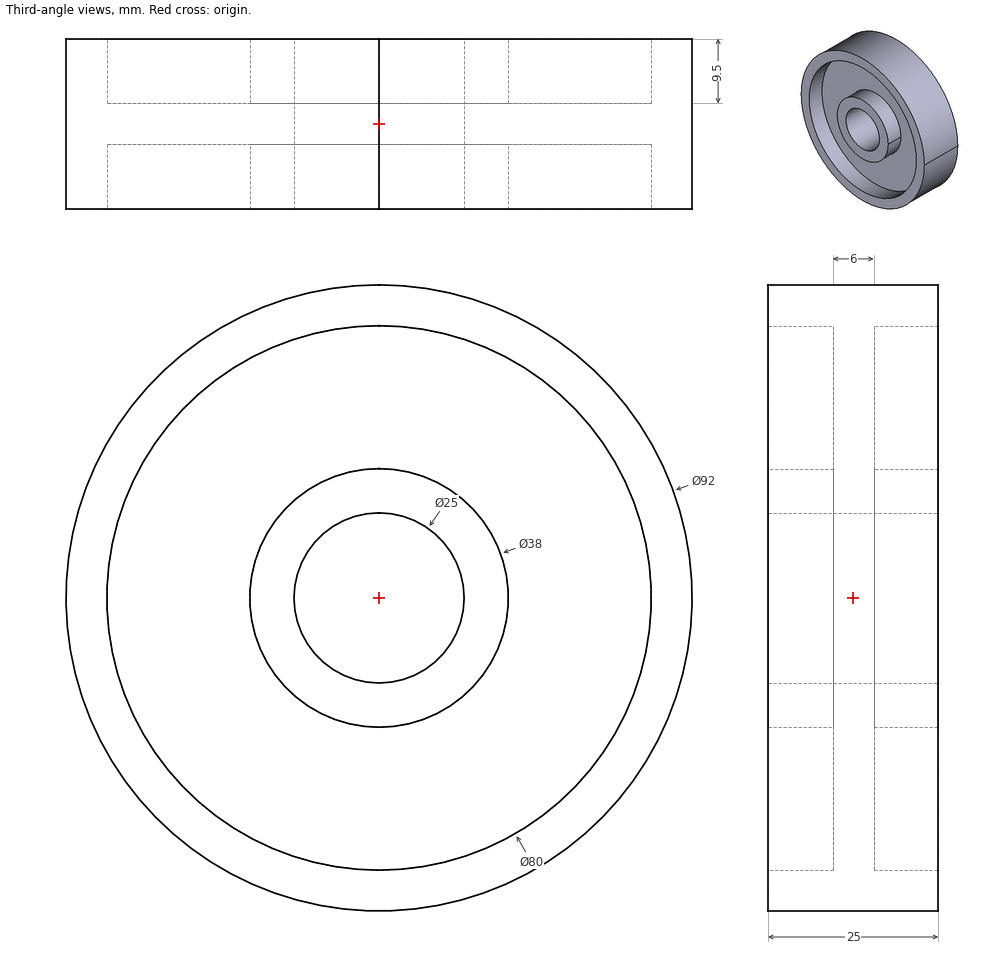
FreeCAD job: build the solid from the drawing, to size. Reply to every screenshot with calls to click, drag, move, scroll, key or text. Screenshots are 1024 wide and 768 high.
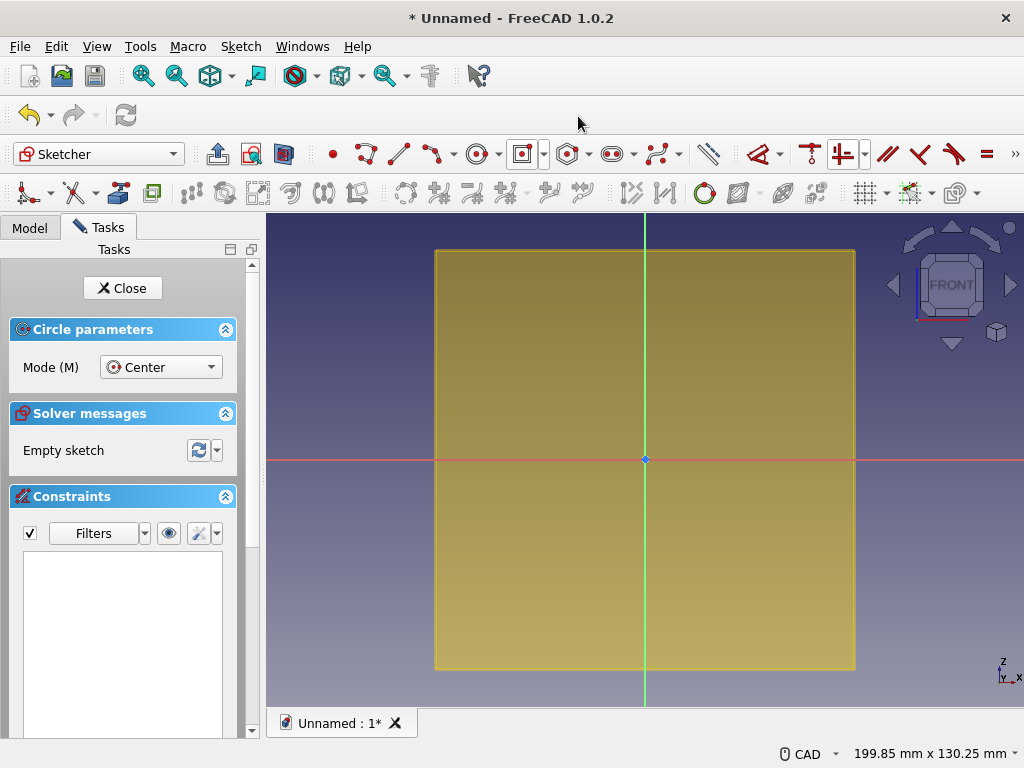
click(645, 460)
move(768, 337)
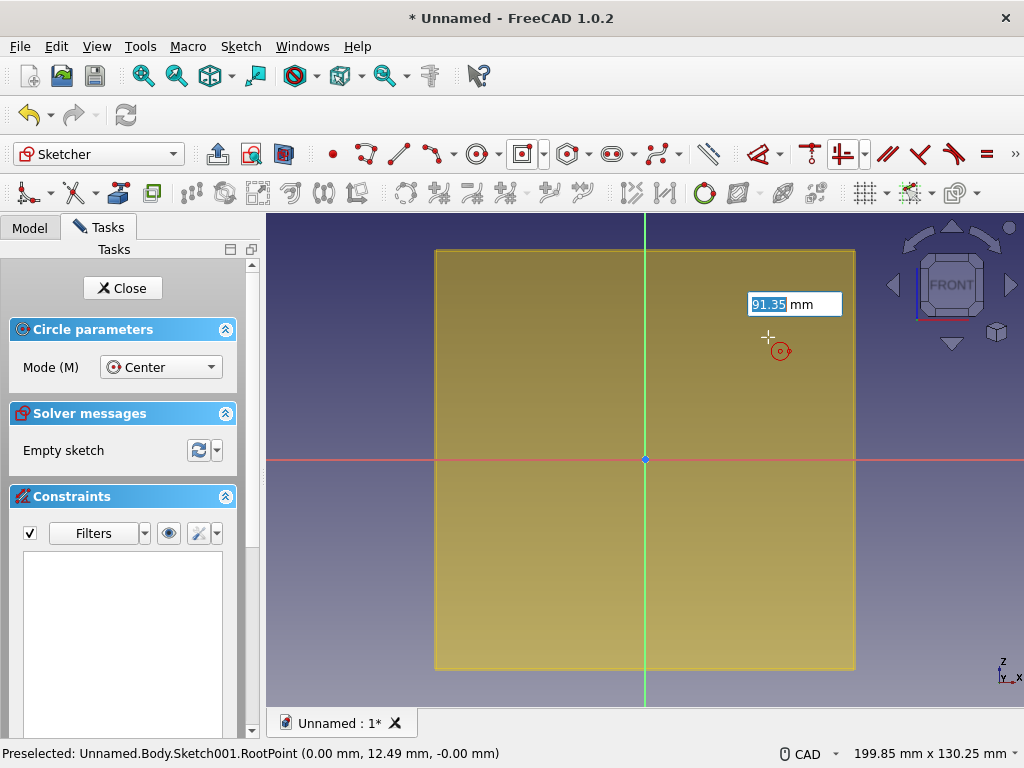
text(92)
key(Return)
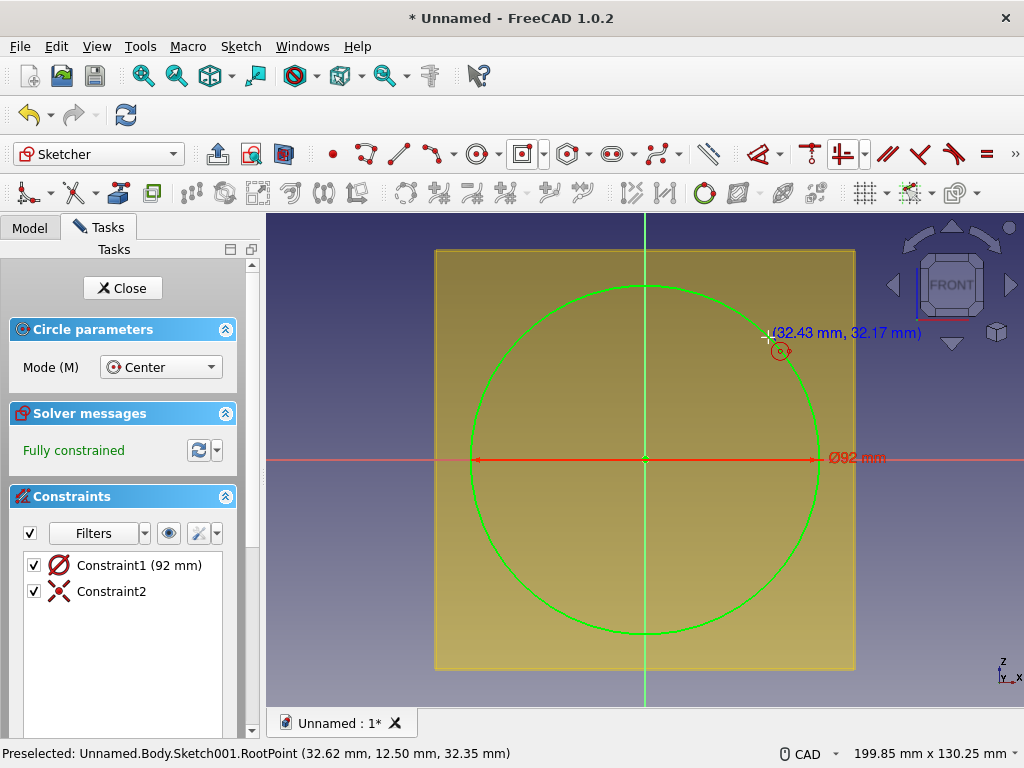
click(645, 460)
move(752, 353)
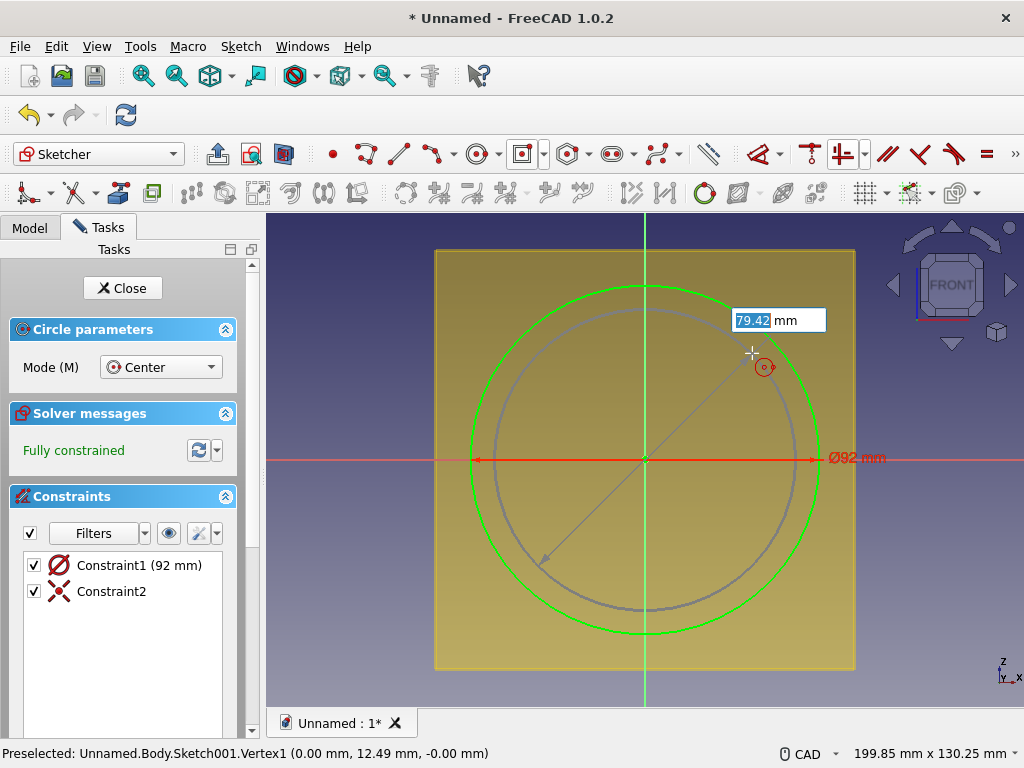
text(80)
key(Return)
key(Escape)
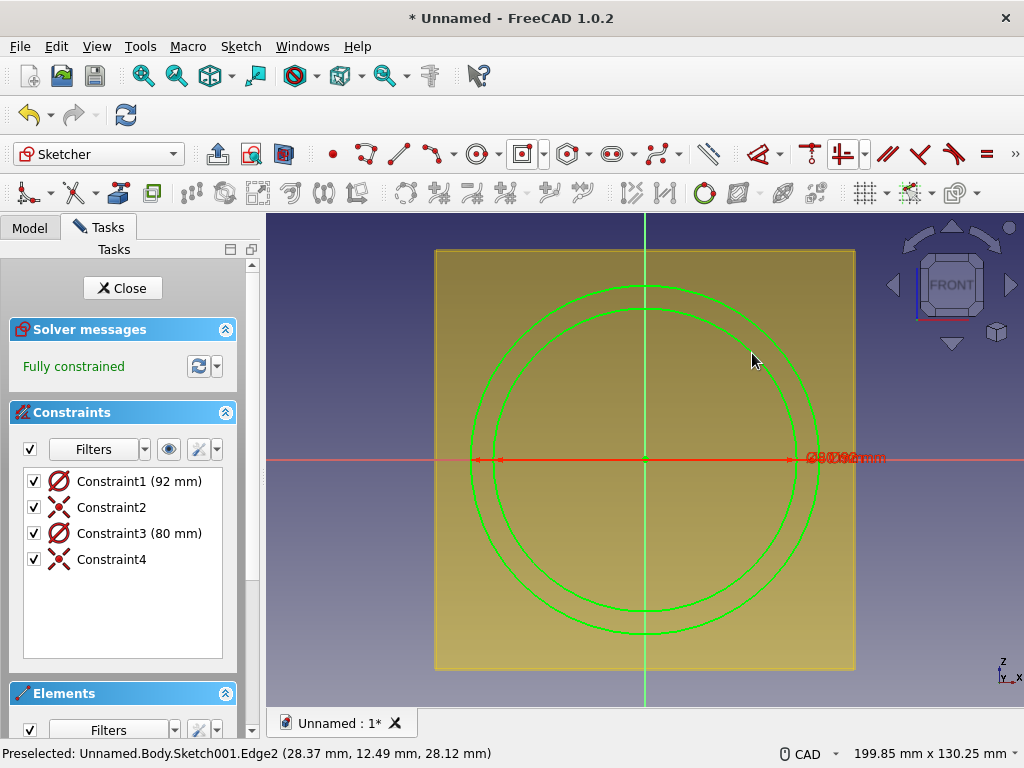
click(123, 288)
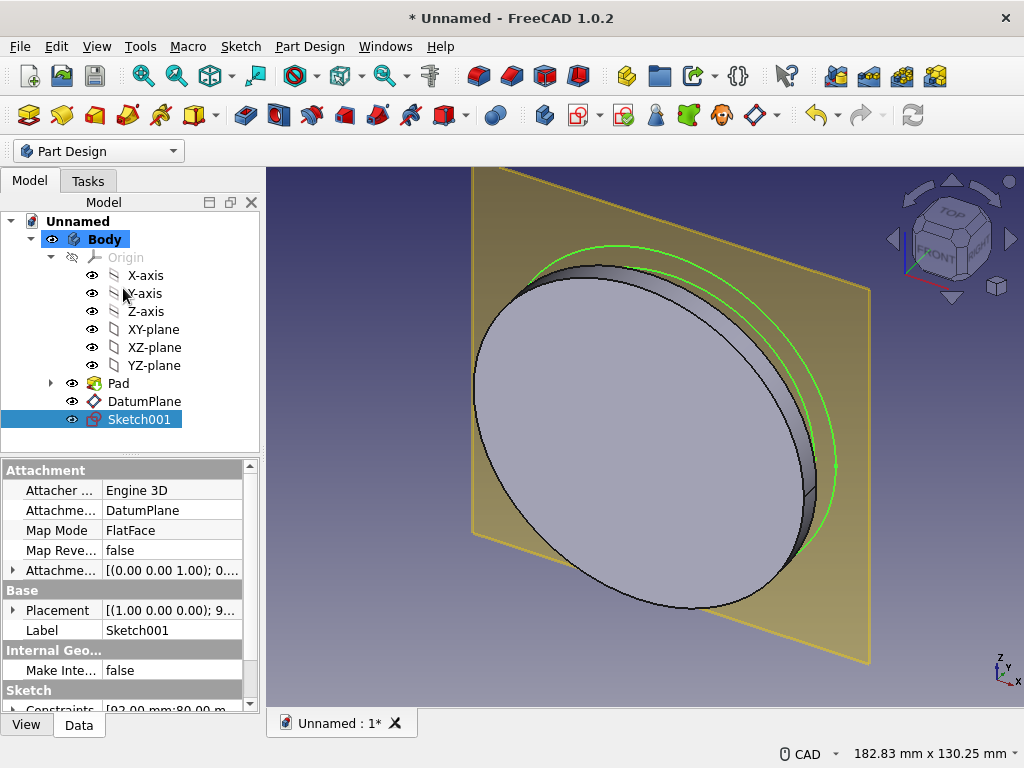
click(29, 116)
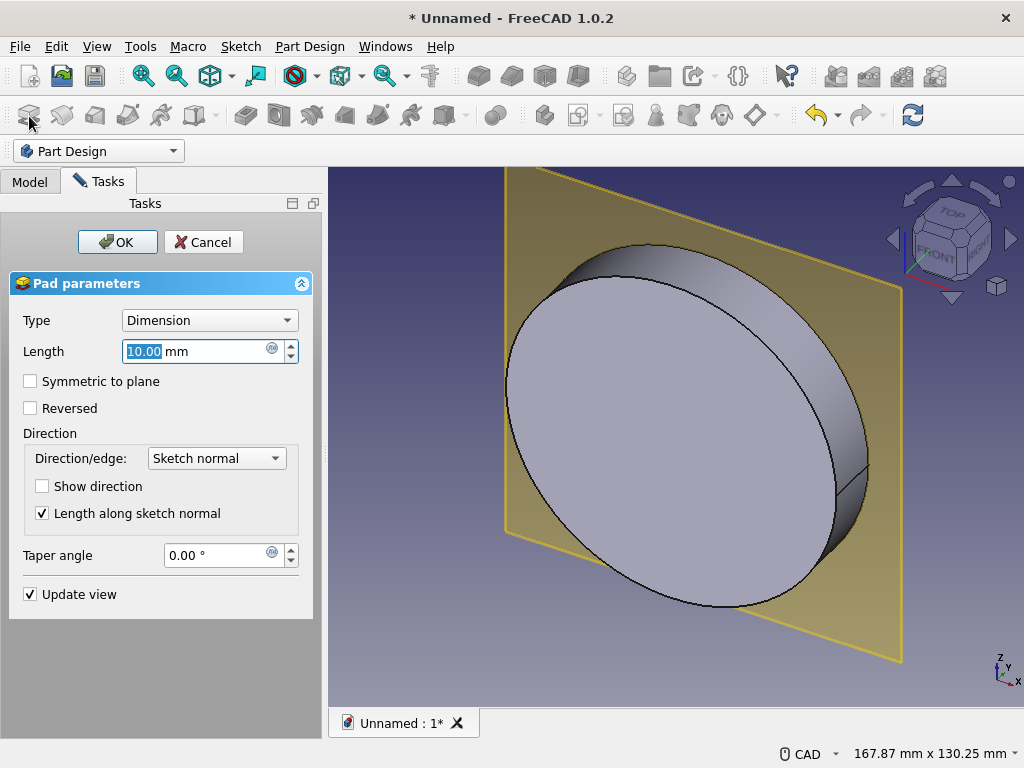
text(9.5)
key(Tab)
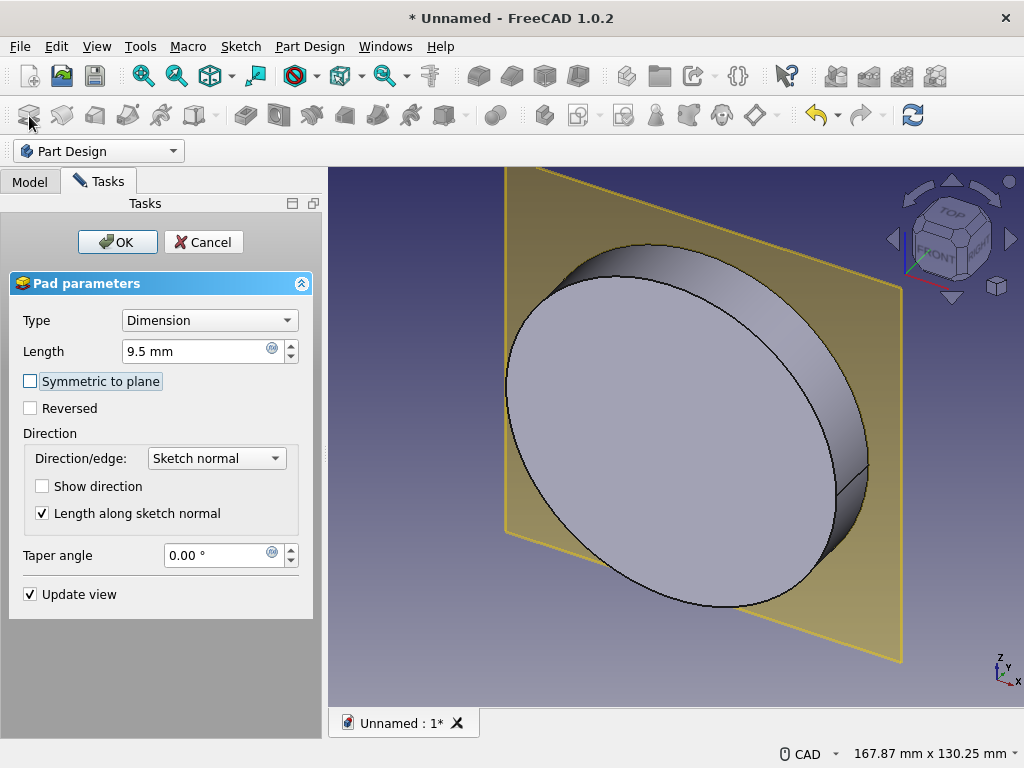
click(118, 242)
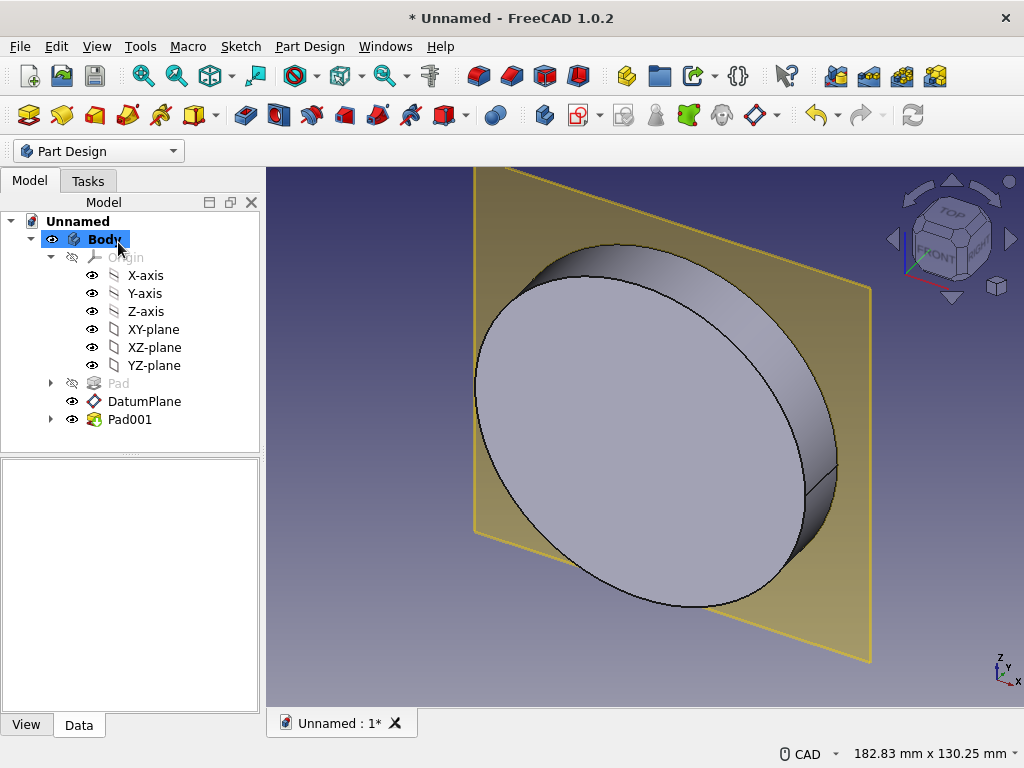
click(117, 401)
key(space)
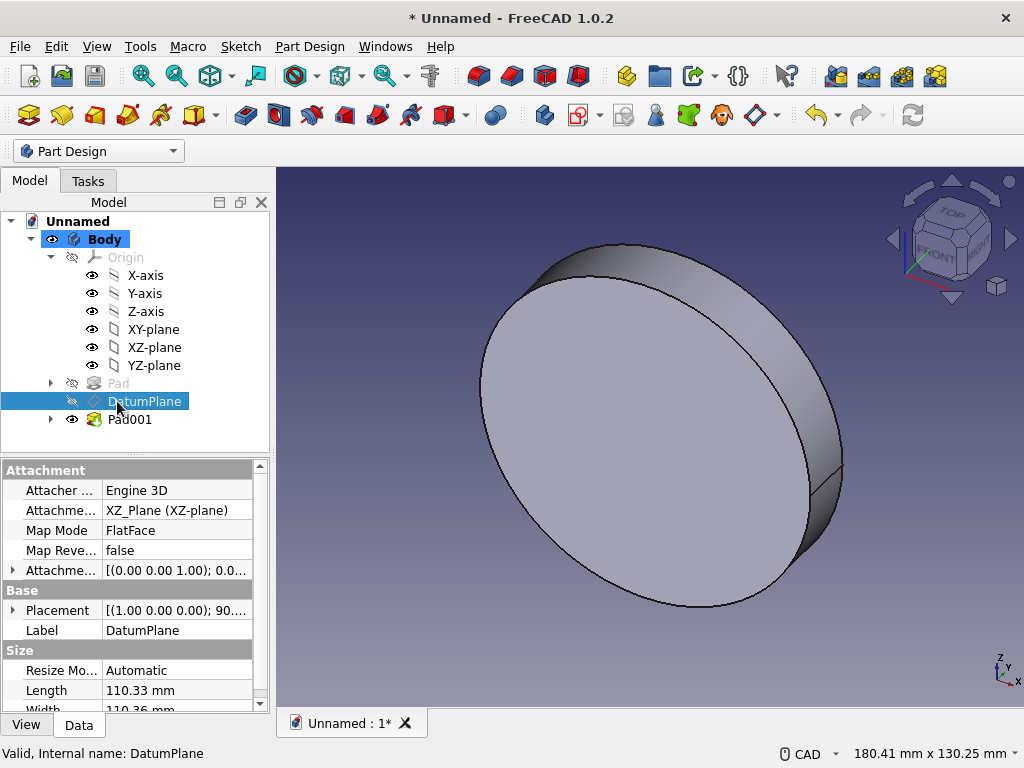
click(117, 419)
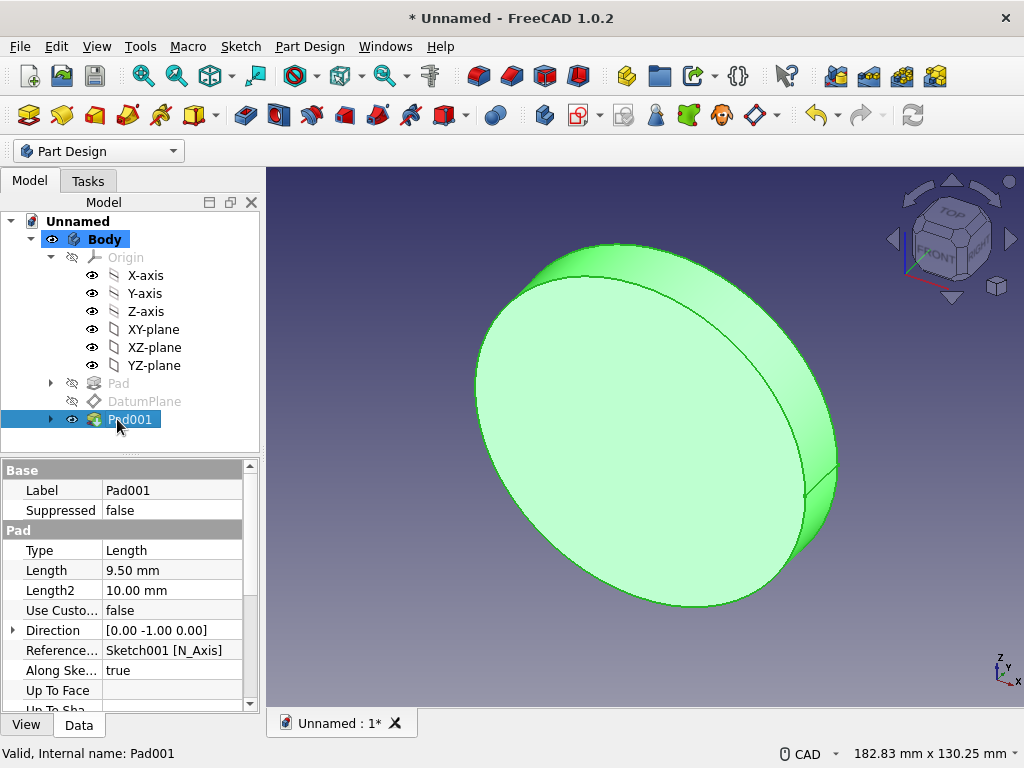
click(836, 76)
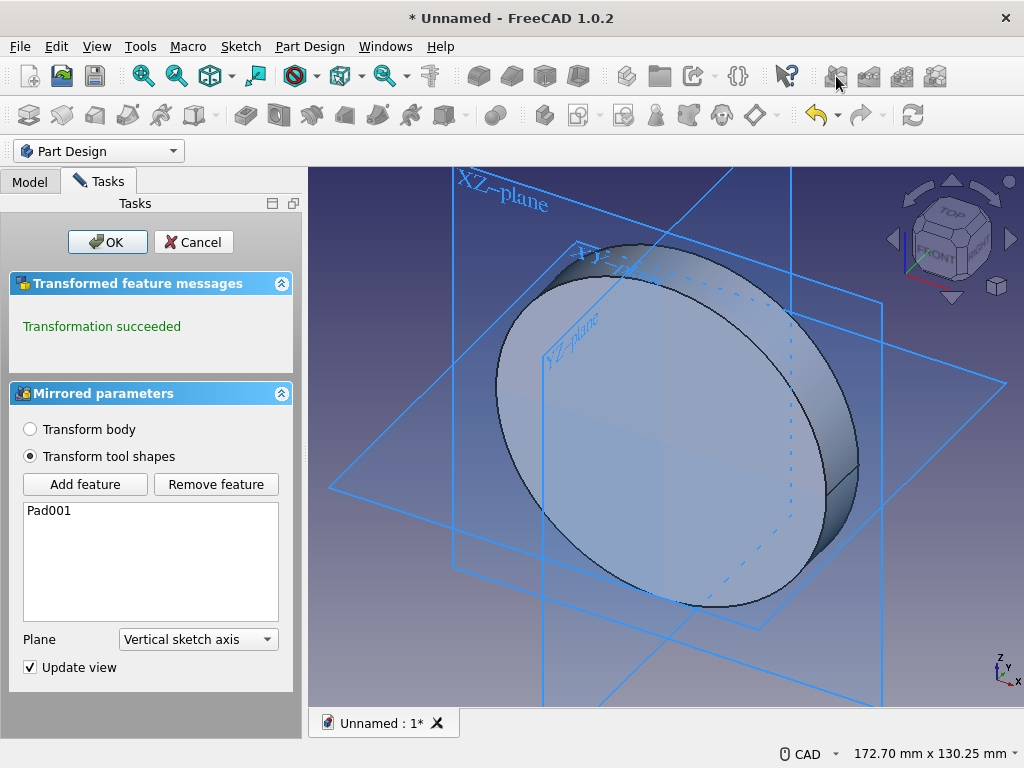
click(199, 640)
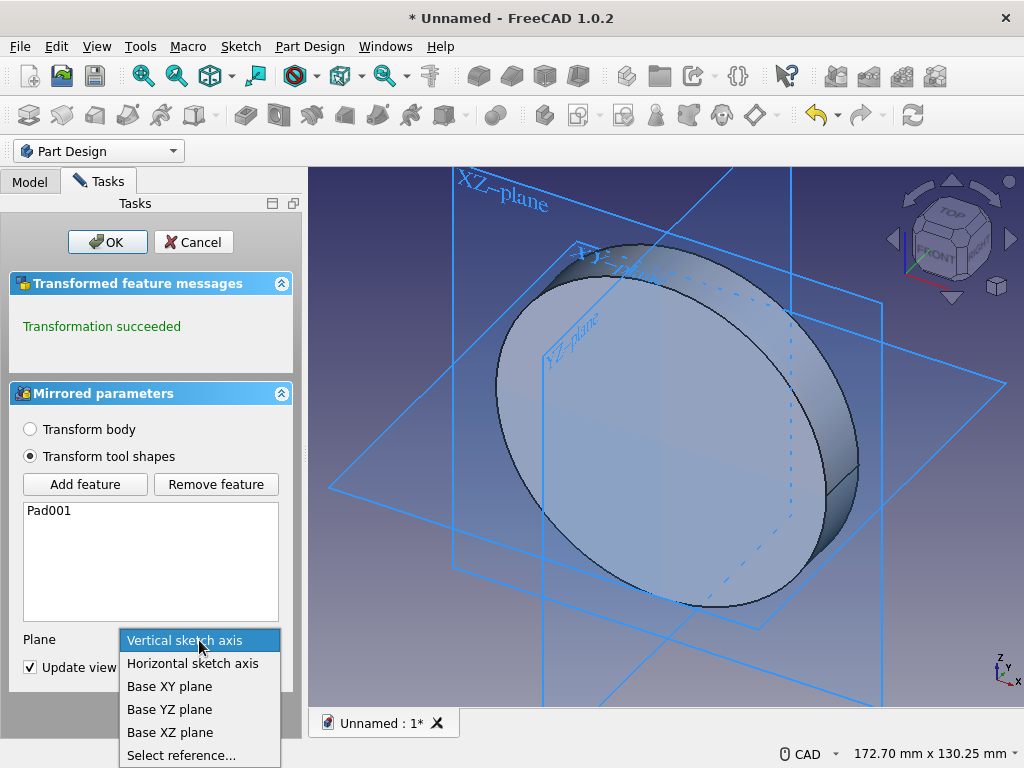
click(198, 732)